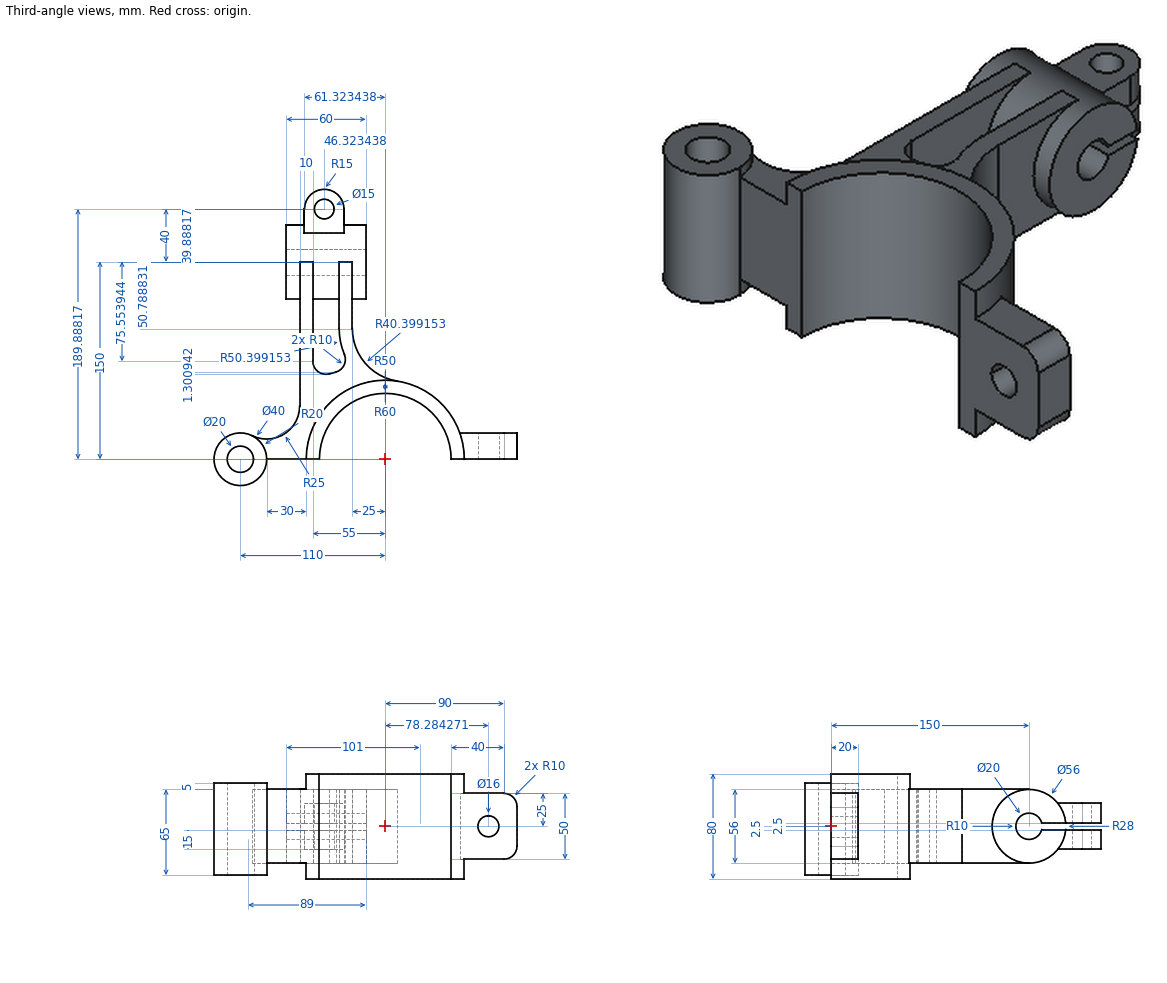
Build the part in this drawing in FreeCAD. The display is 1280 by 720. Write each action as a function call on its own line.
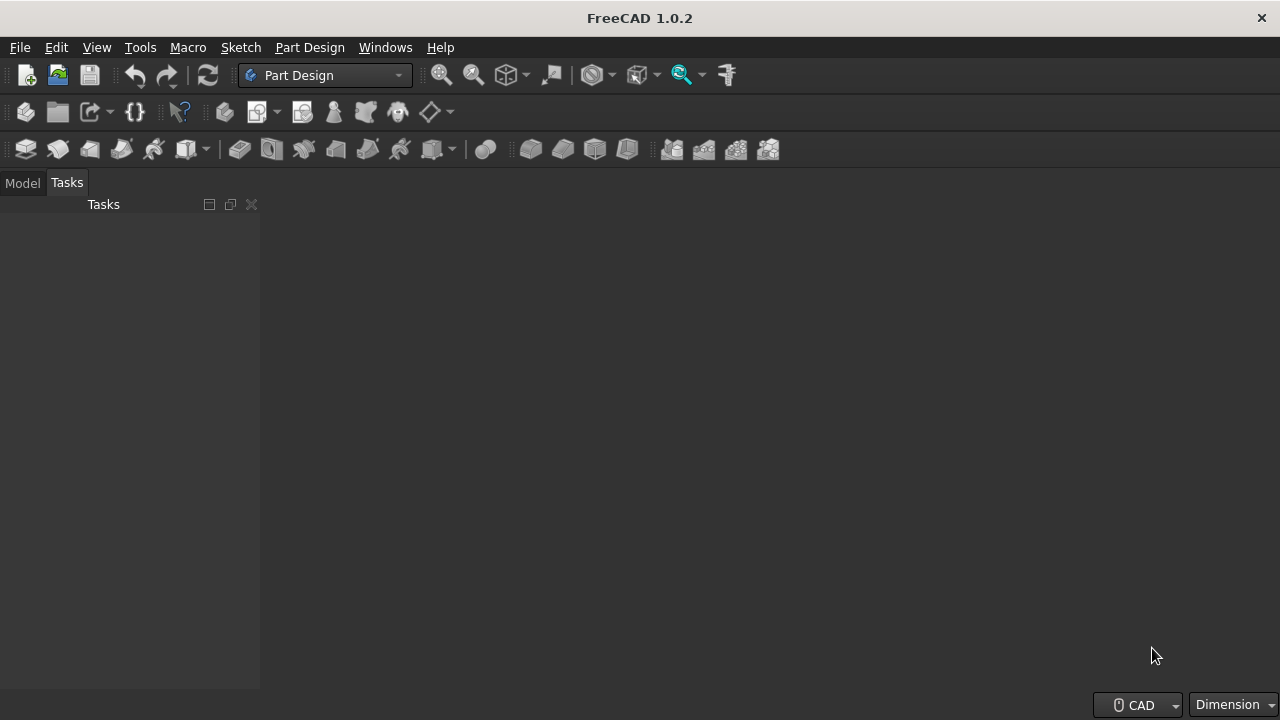
key(ctrl+n)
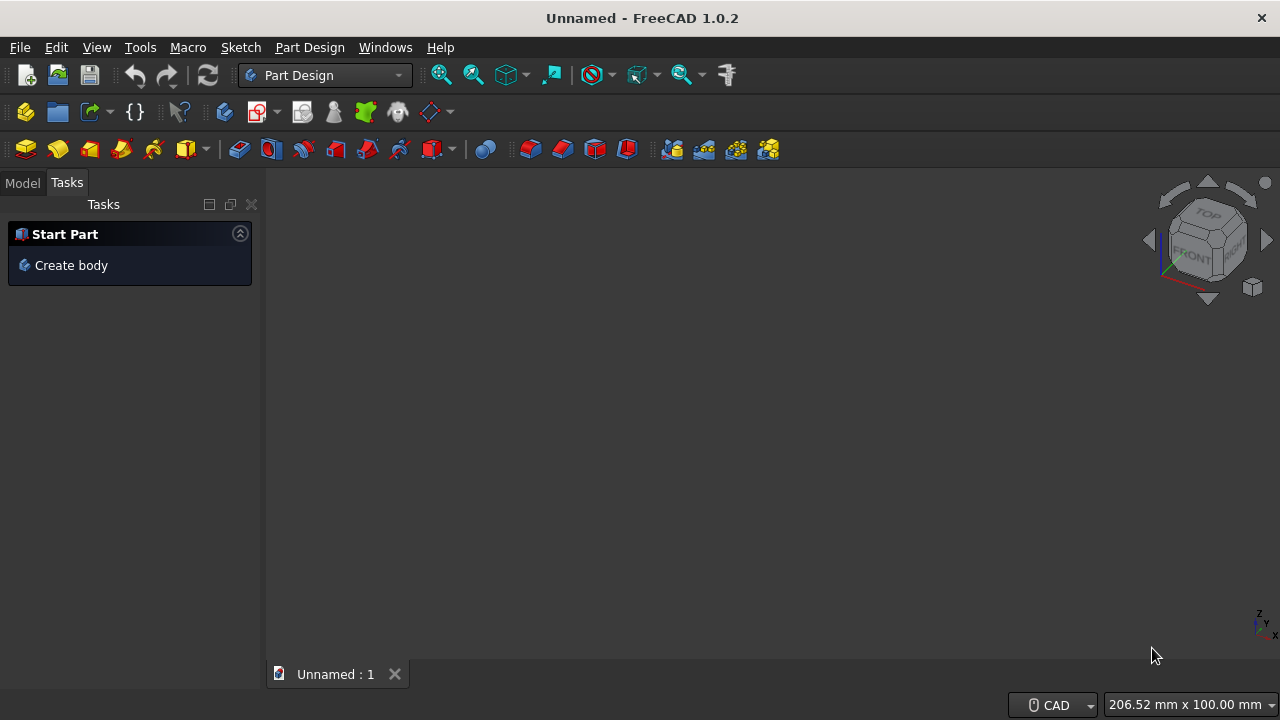
click(258, 112)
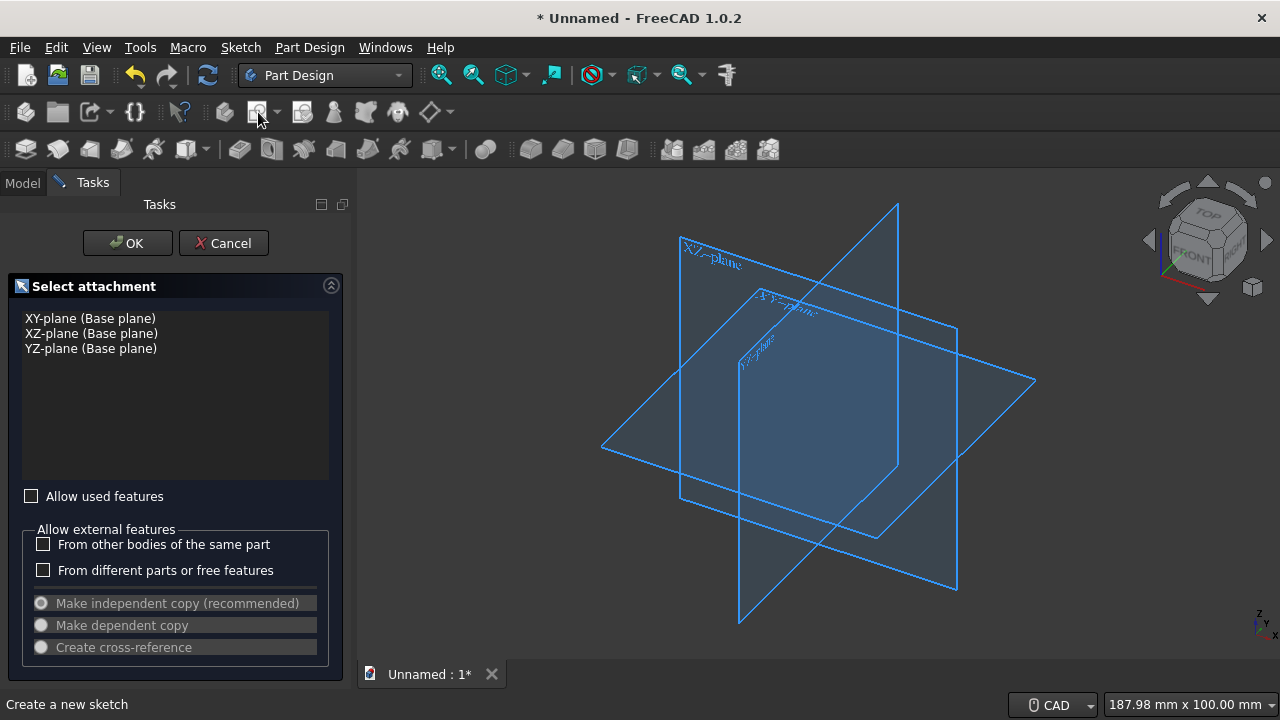
click(82, 318)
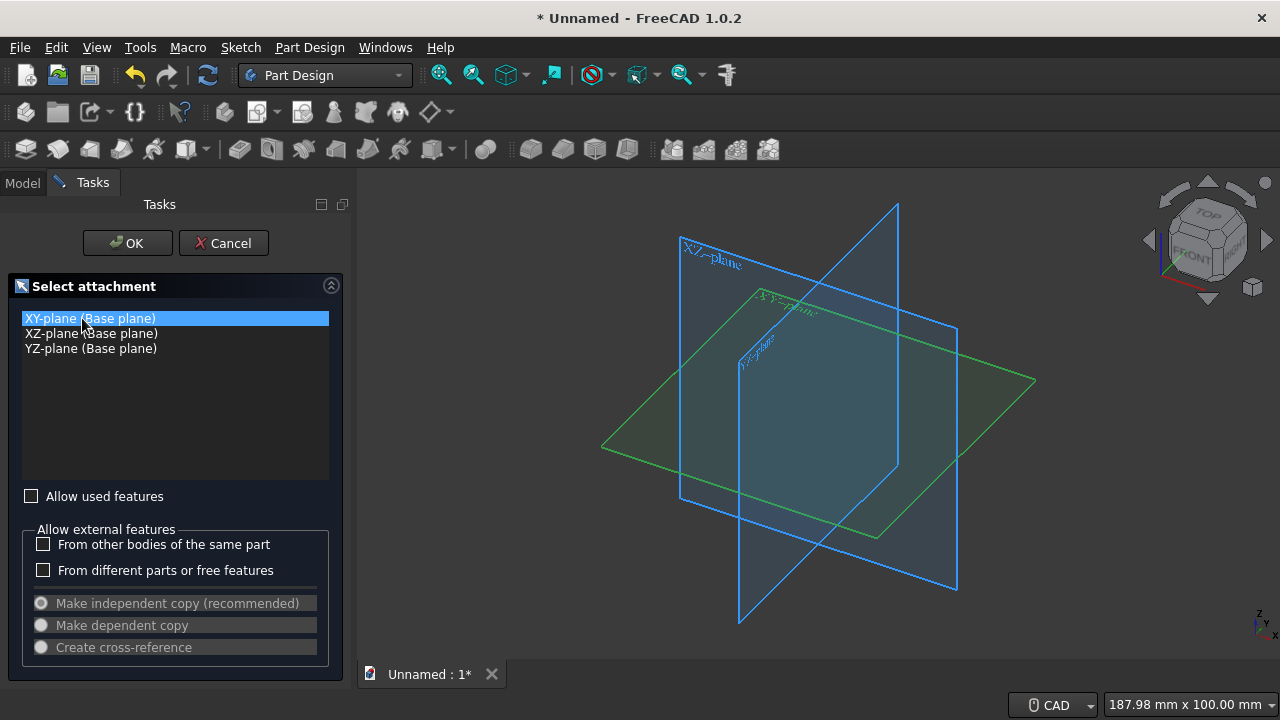
click(128, 243)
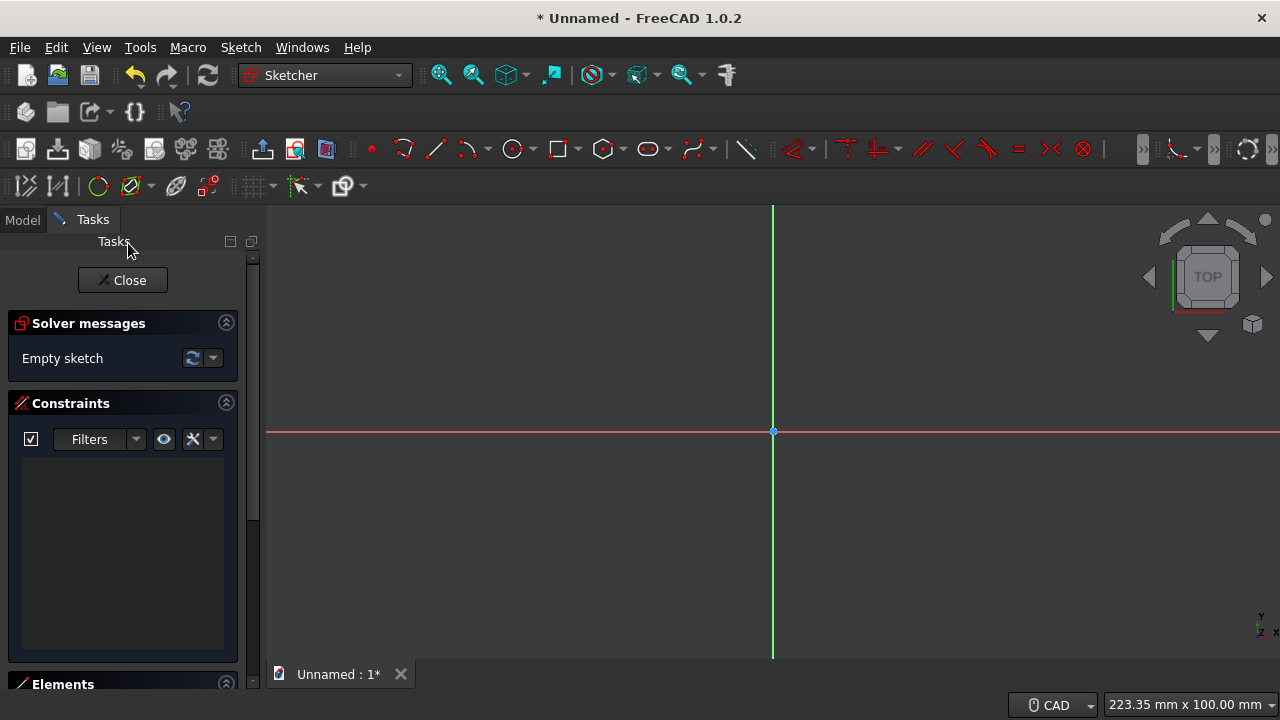
scroll(565, 631, down, 2)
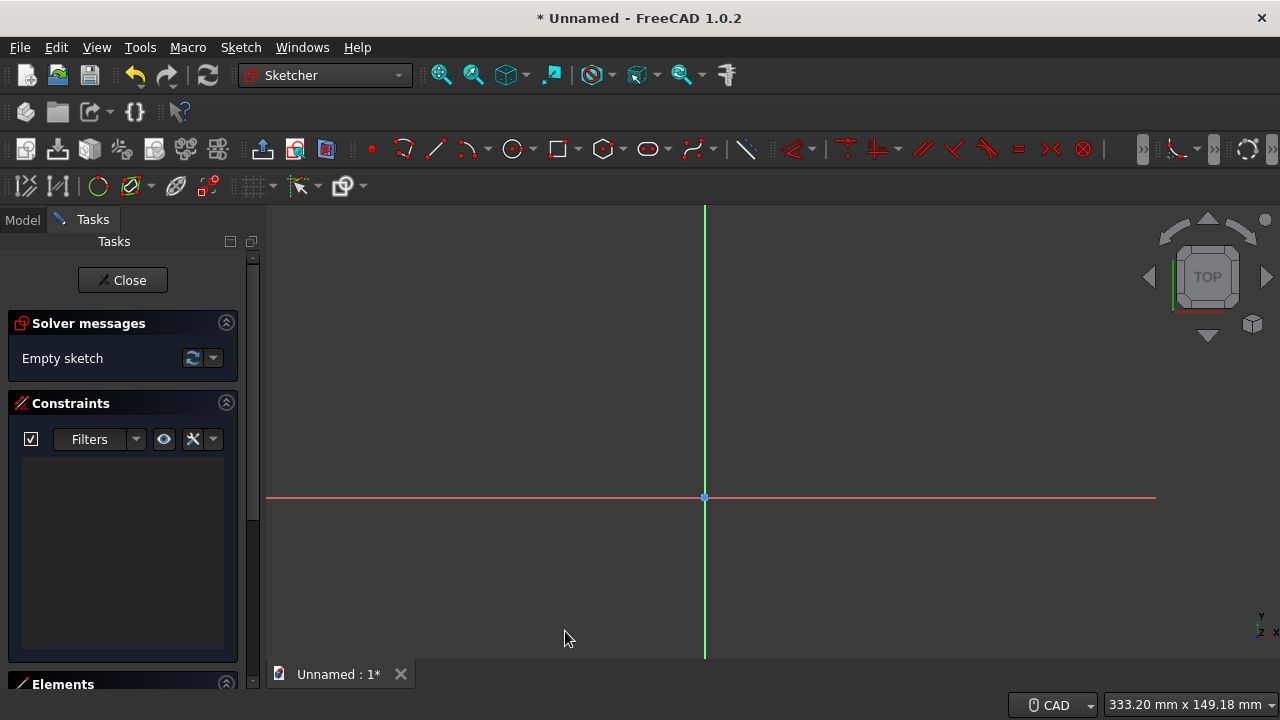
scroll(705, 355, up, 2)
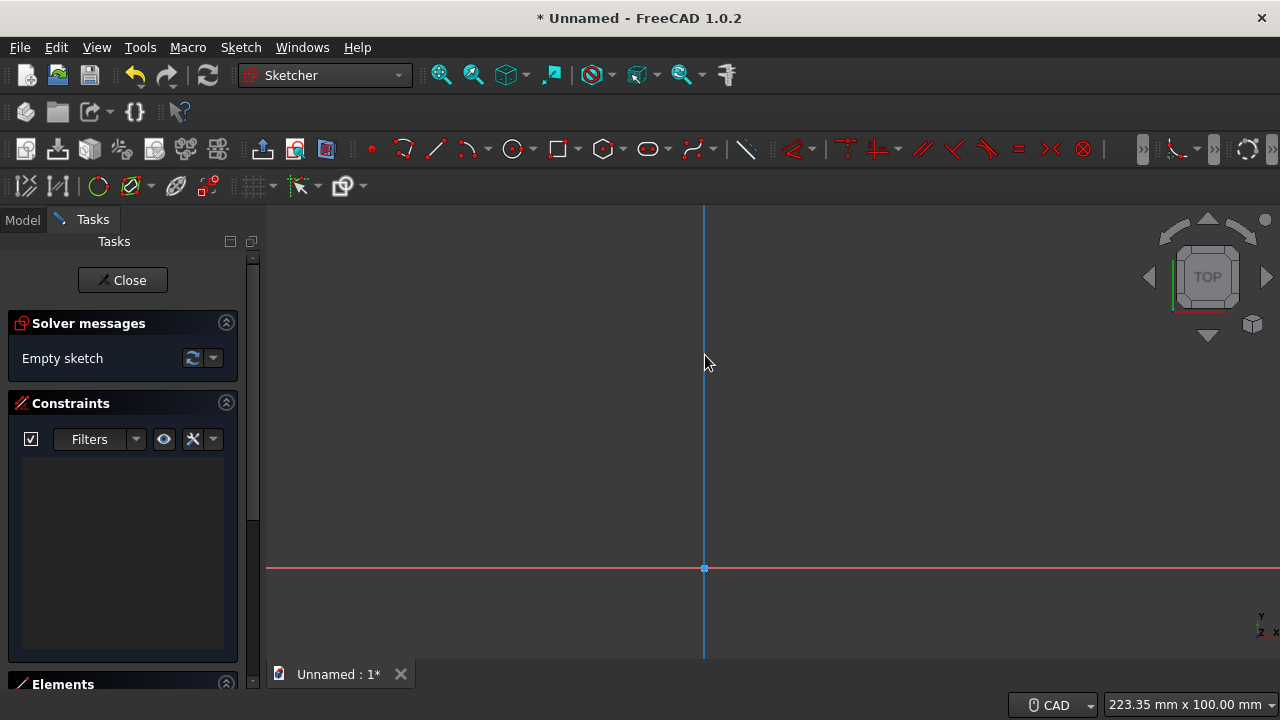
key(g)
key(l)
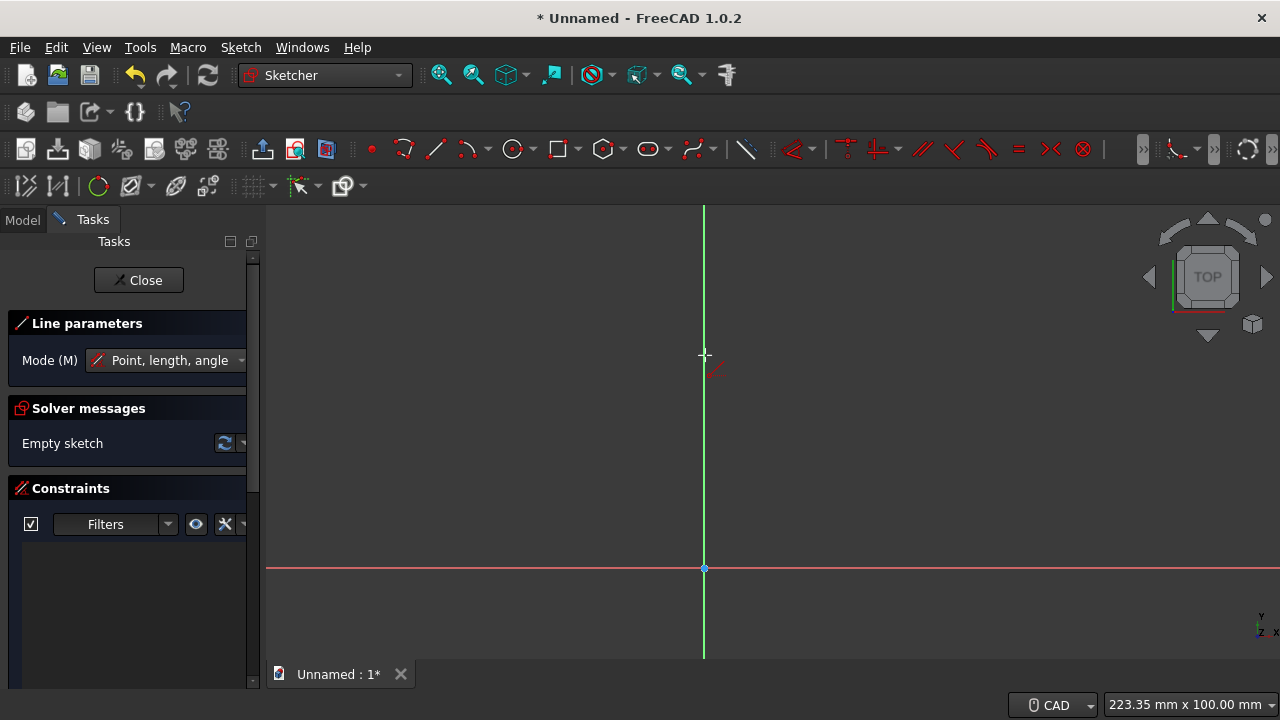
click(432, 568)
click(477, 559)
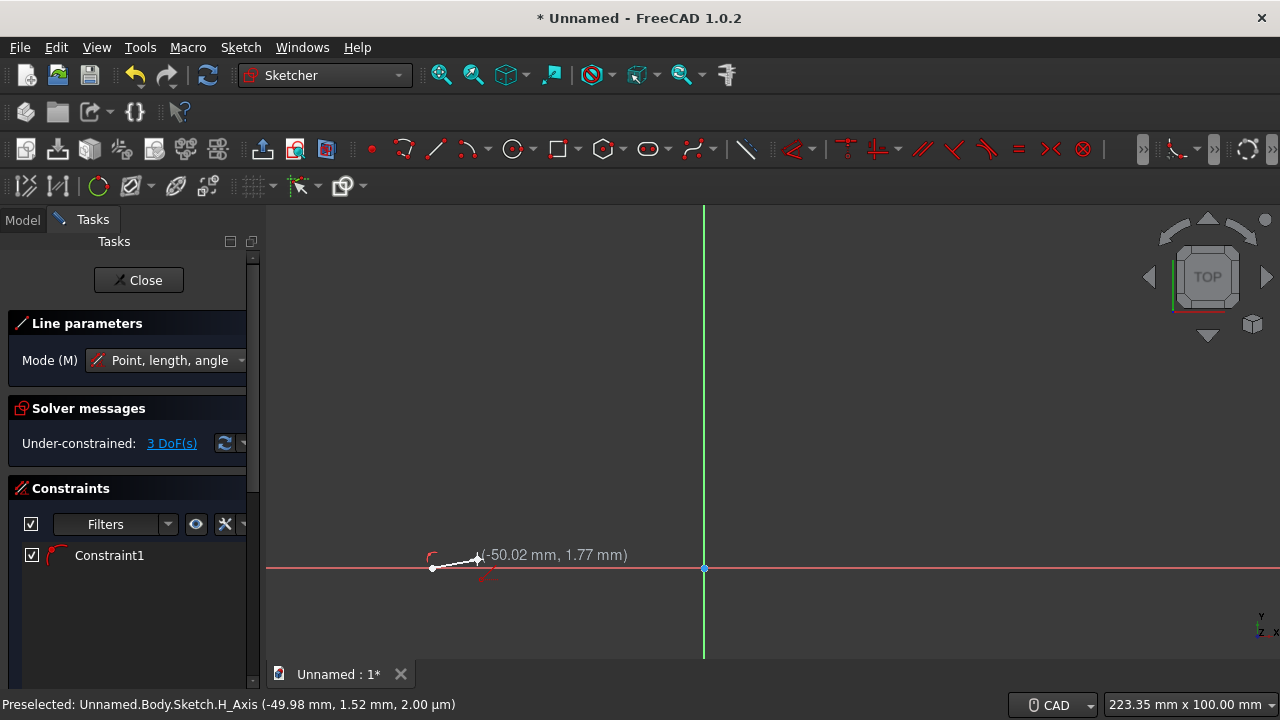
click(931, 568)
click(976, 559)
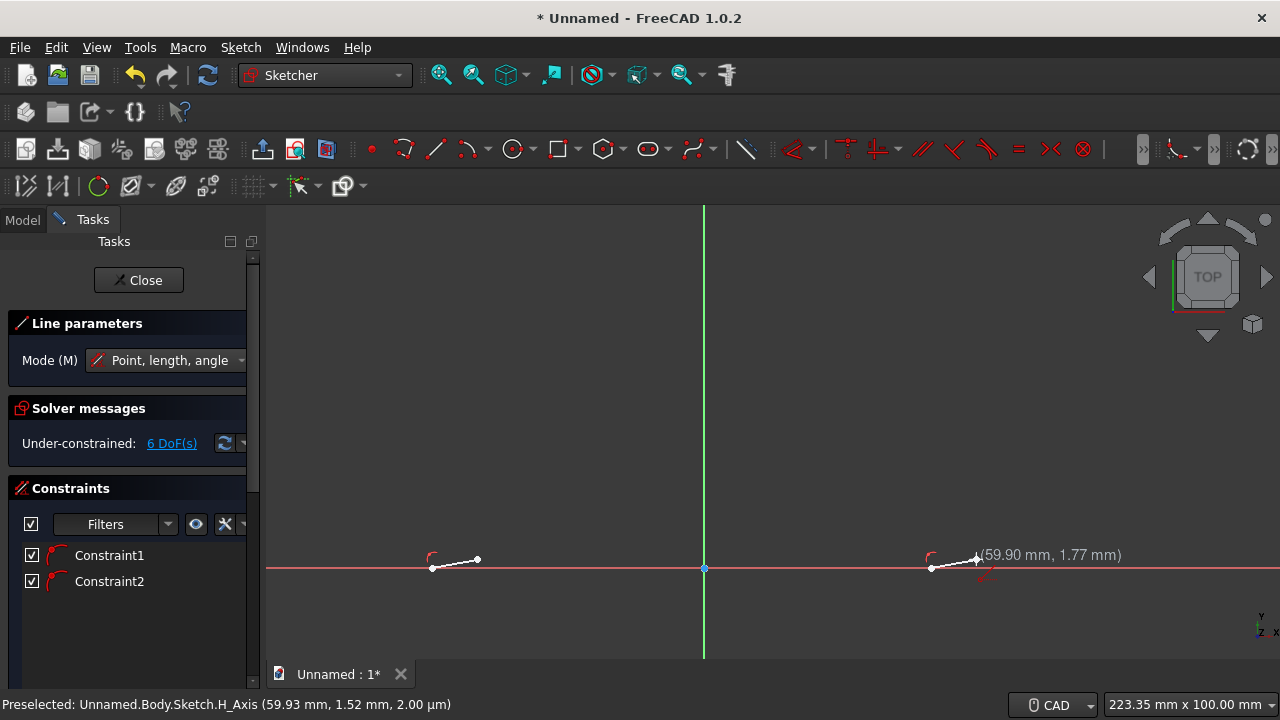
key(g)
key(3)
key(a)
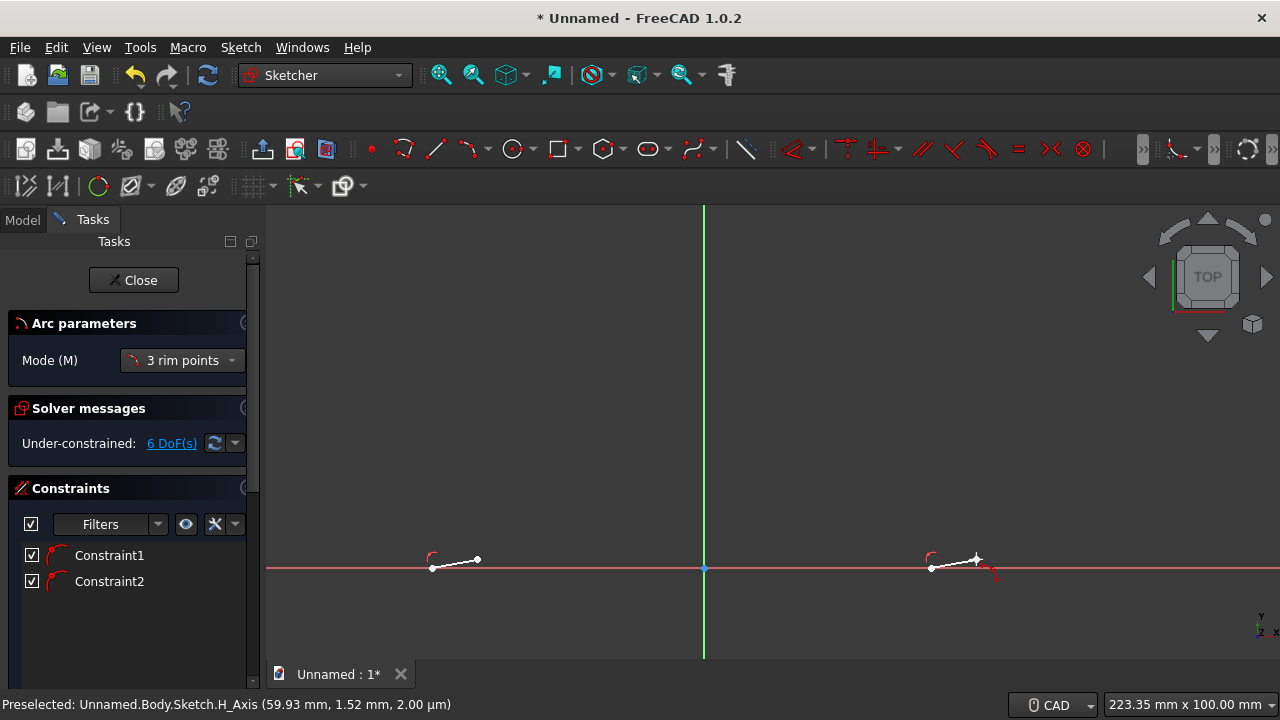
click(477, 560)
click(931, 568)
click(774, 352)